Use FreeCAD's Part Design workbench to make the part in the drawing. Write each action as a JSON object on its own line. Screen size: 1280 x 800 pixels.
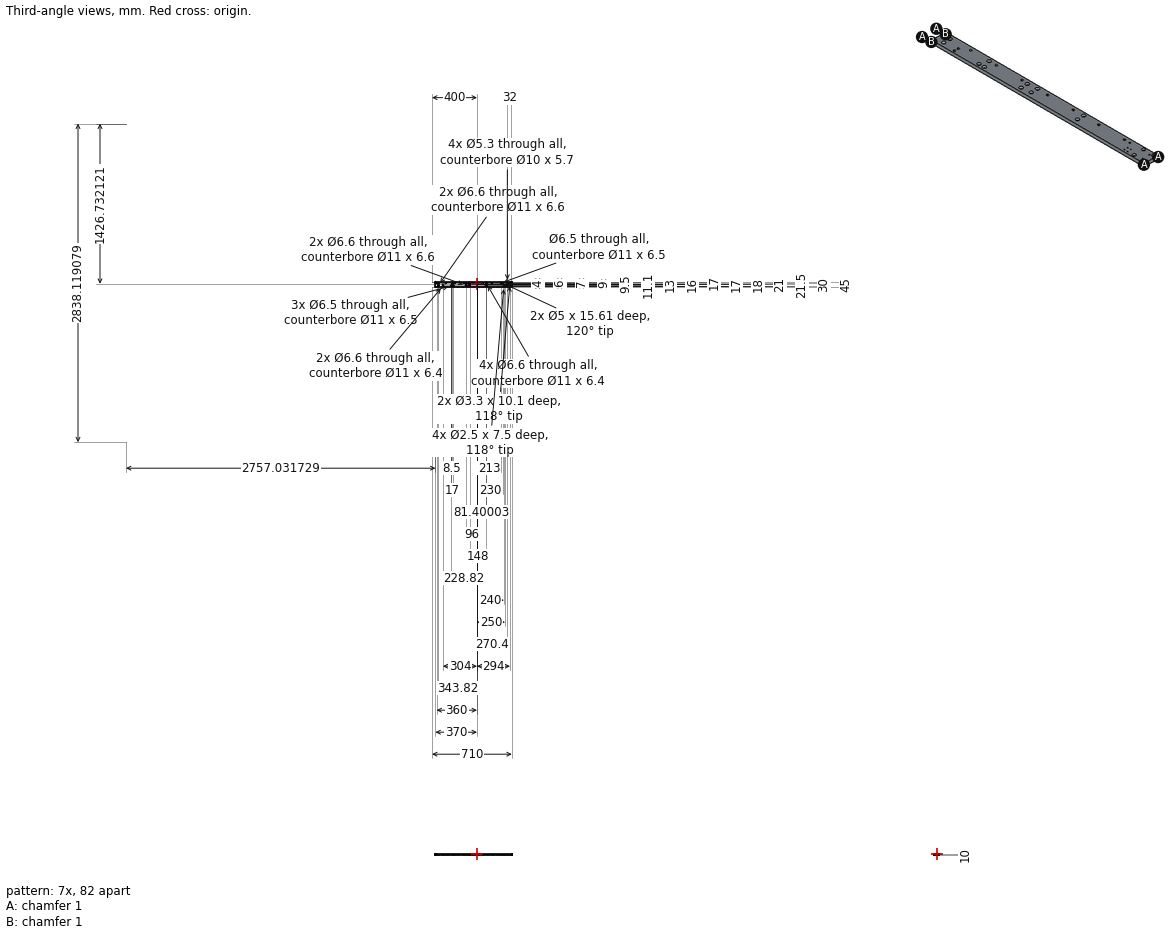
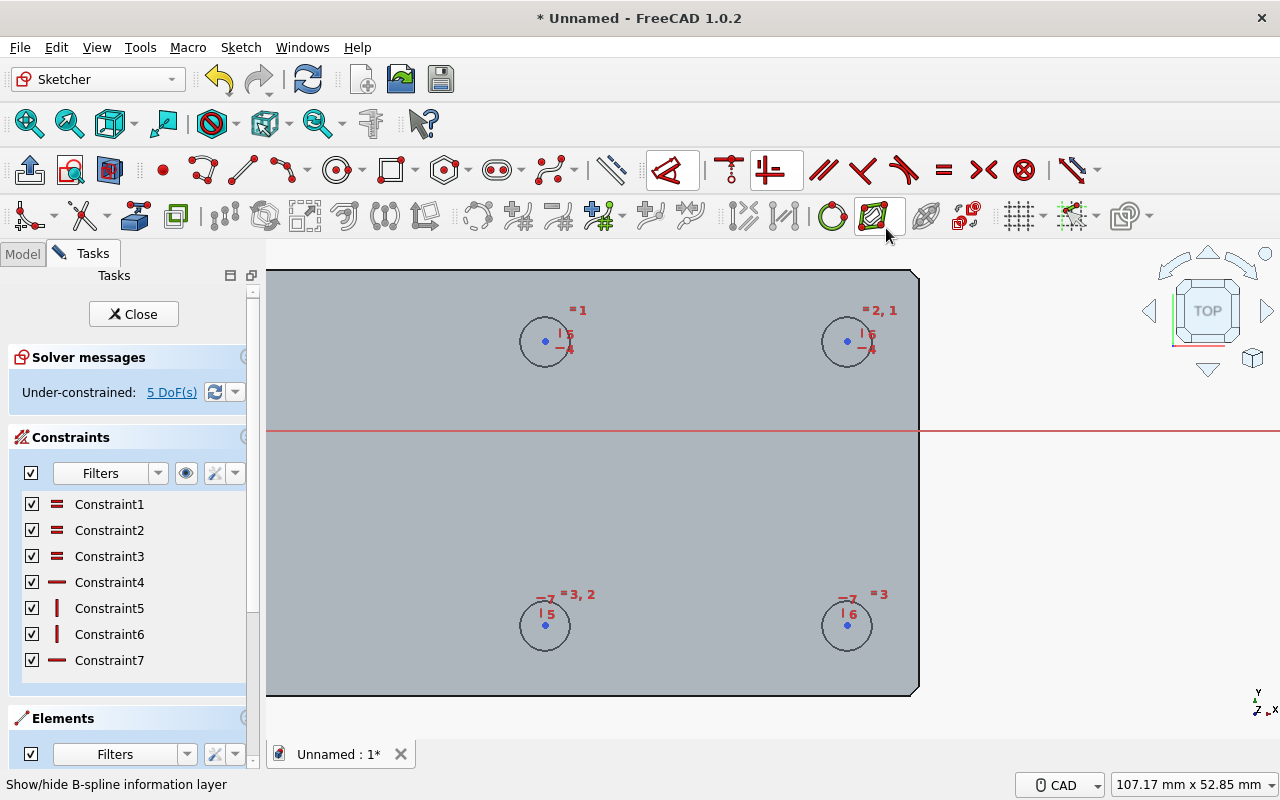
{"action": "left_click", "coordinate": [562, 324]}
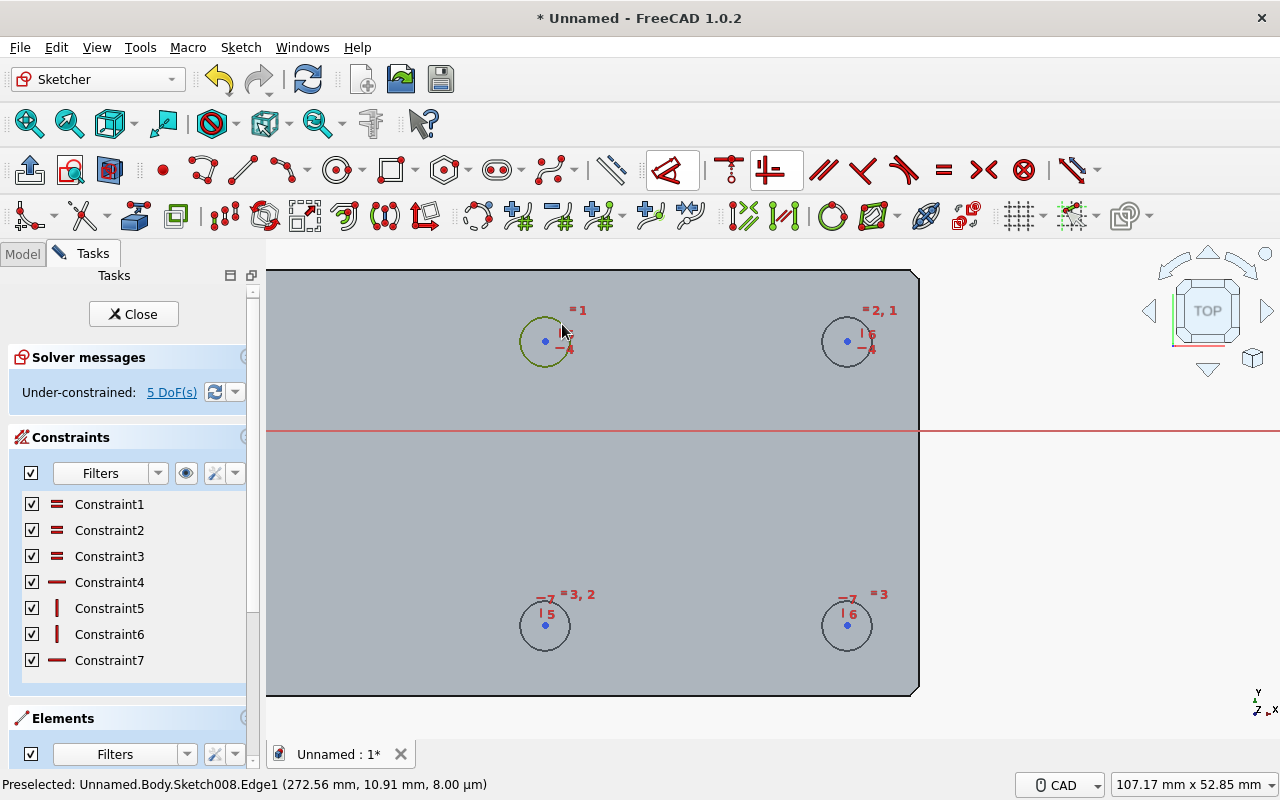
{"action": "key", "text": "k o"}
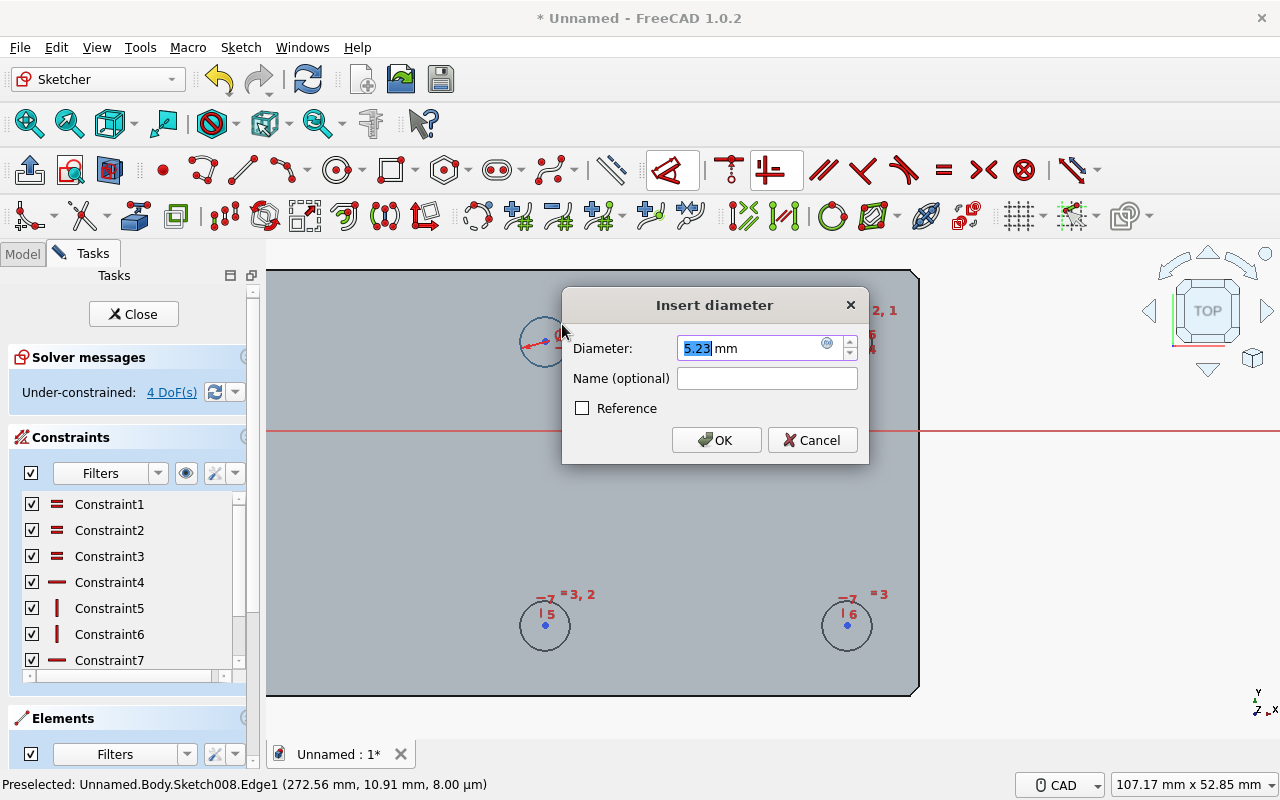
{"action": "type", "text": "5.3"}
{"action": "key", "text": "Return"}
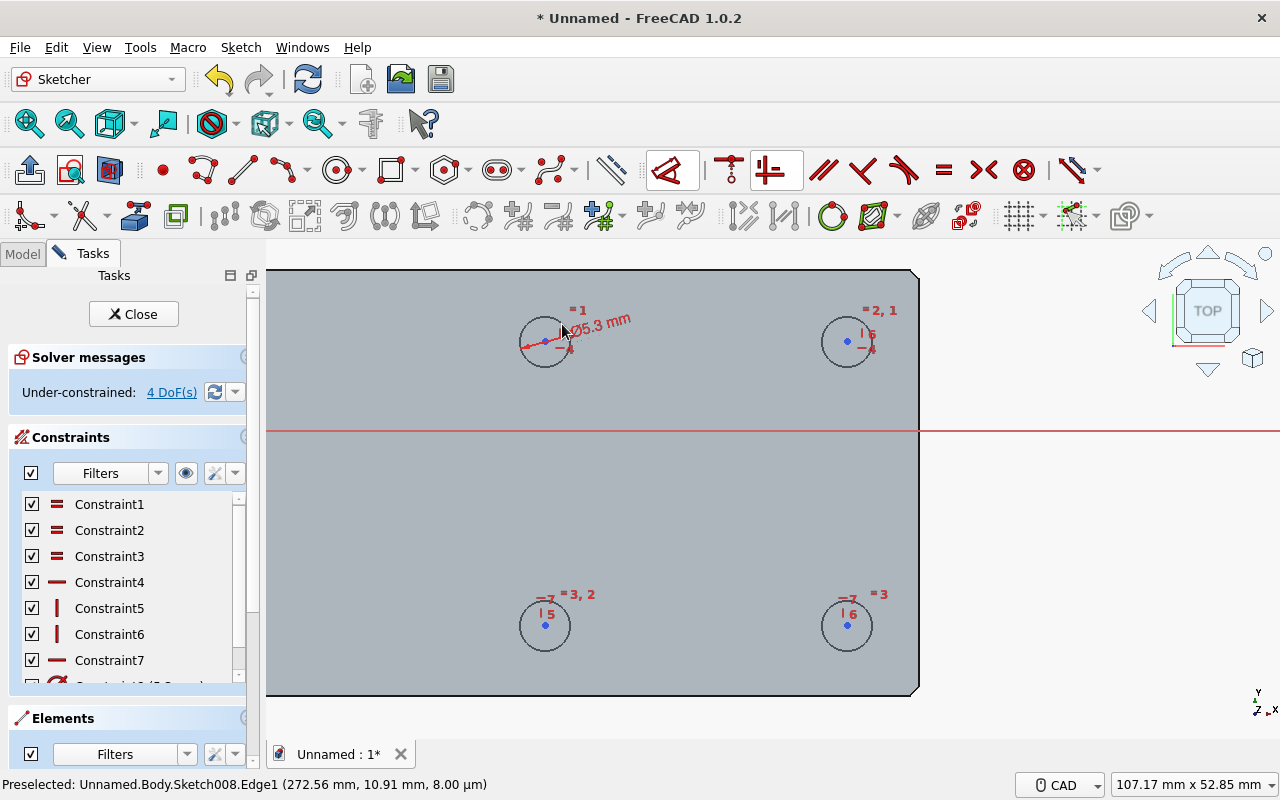
{"action": "left_click", "coordinate": [545, 342]}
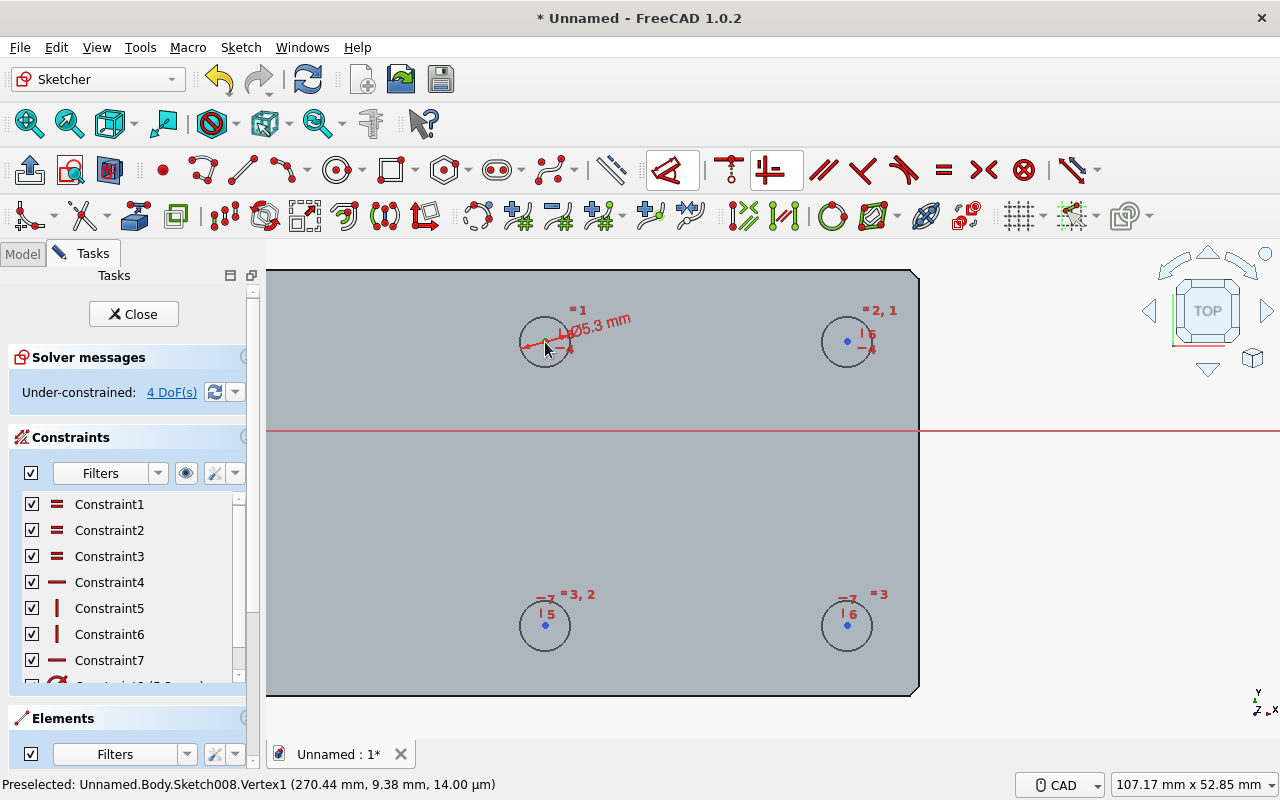
{"action": "left_click", "coordinate": [694, 170]}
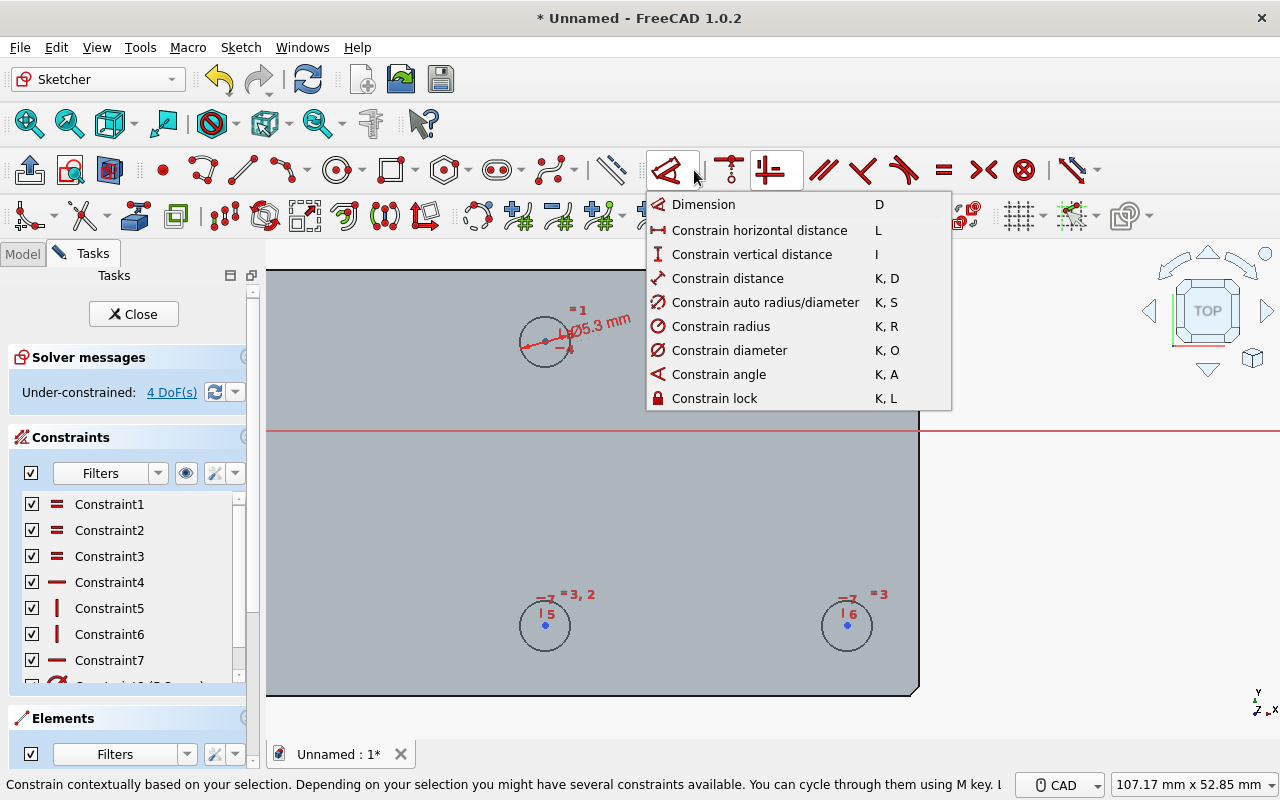
{"action": "left_click", "coordinate": [799, 254]}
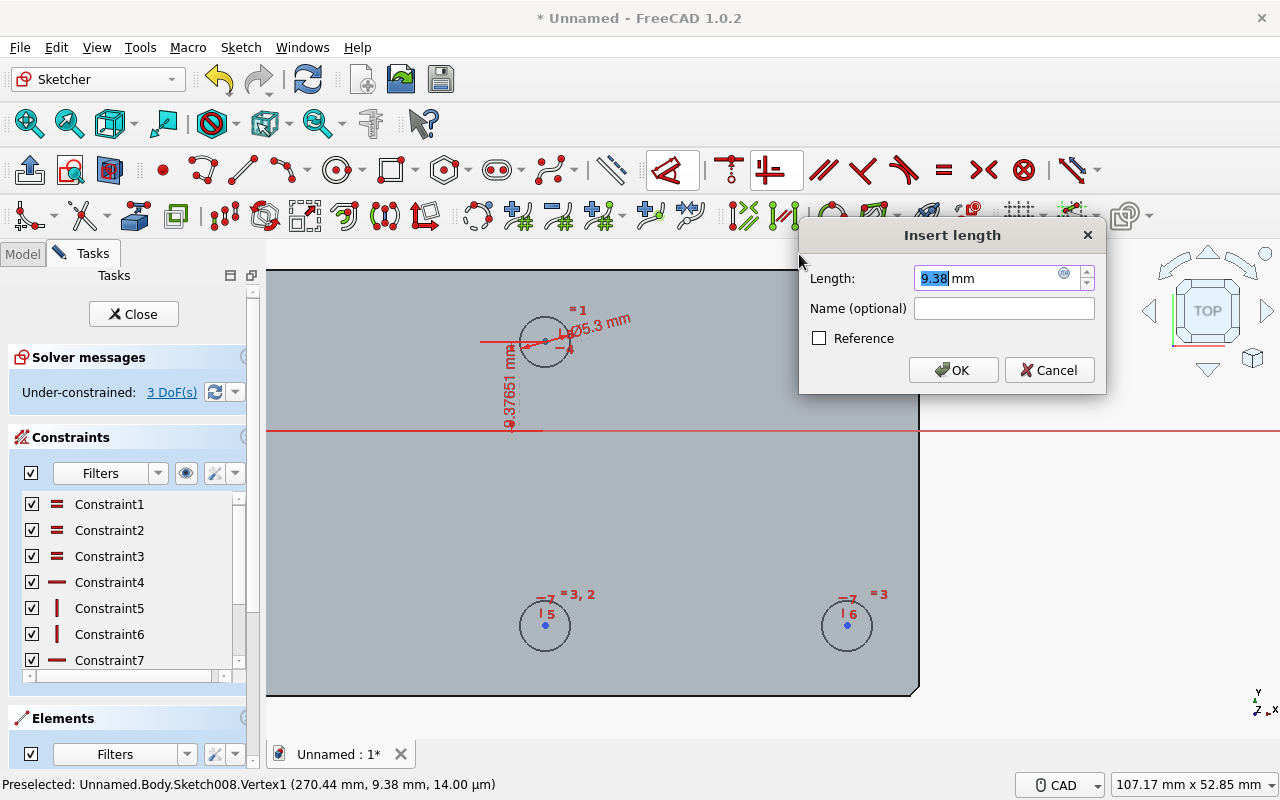
{"action": "type", "text": "9.5"}
{"action": "key", "text": "Return"}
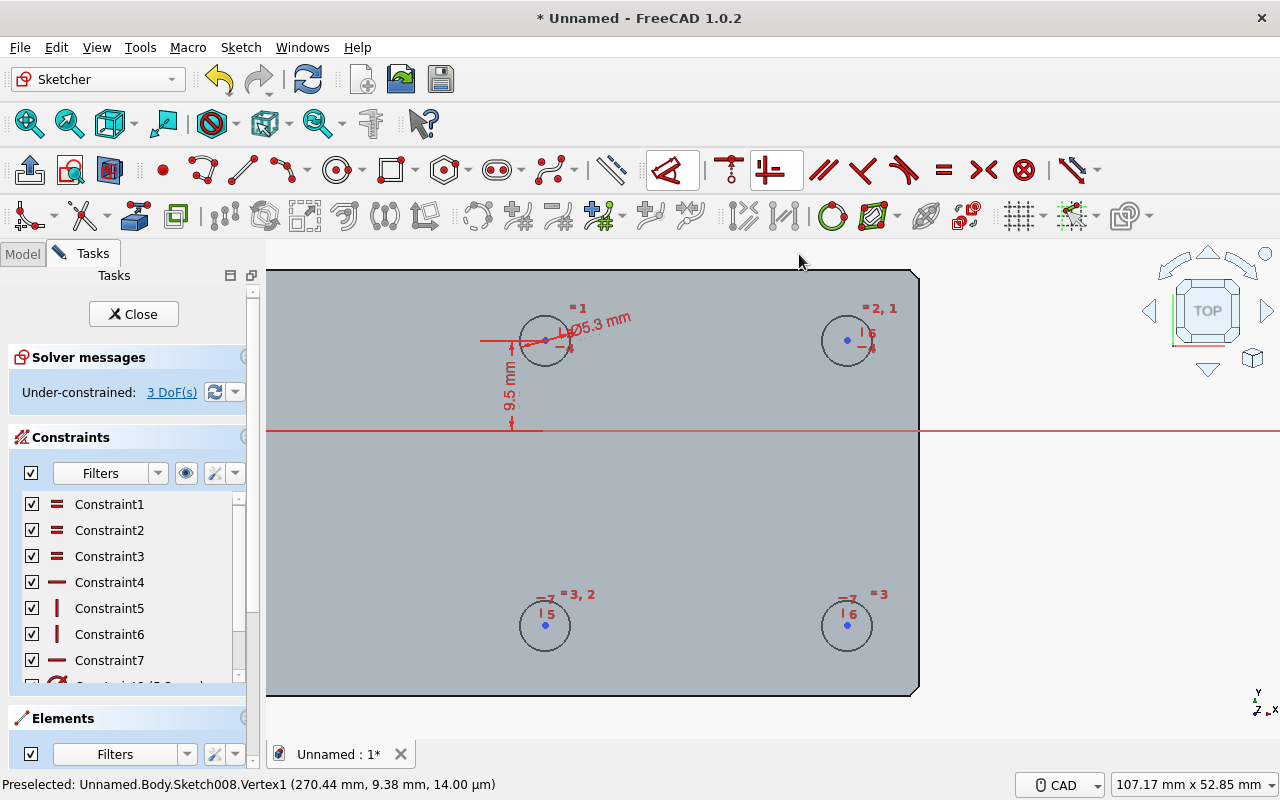
{"action": "left_click", "coordinate": [545, 341]}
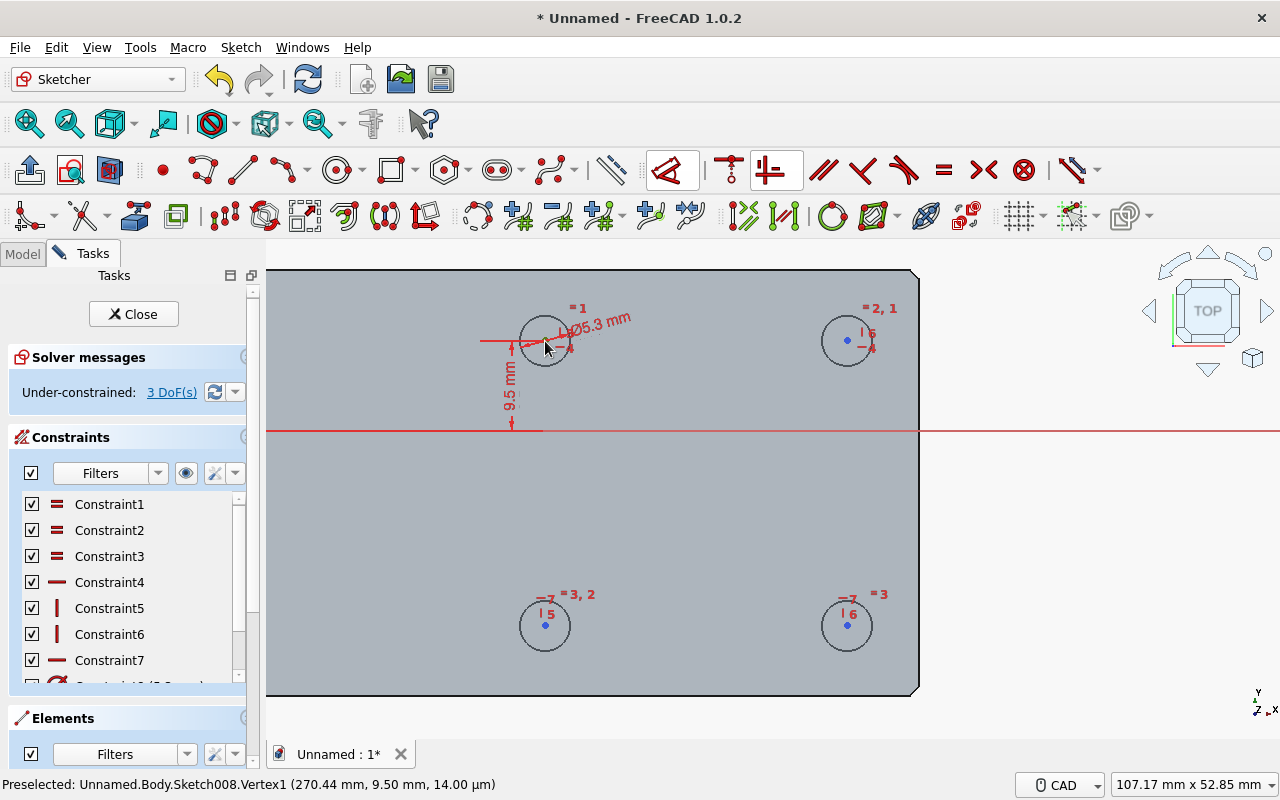
{"action": "left_click", "coordinate": [847, 341]}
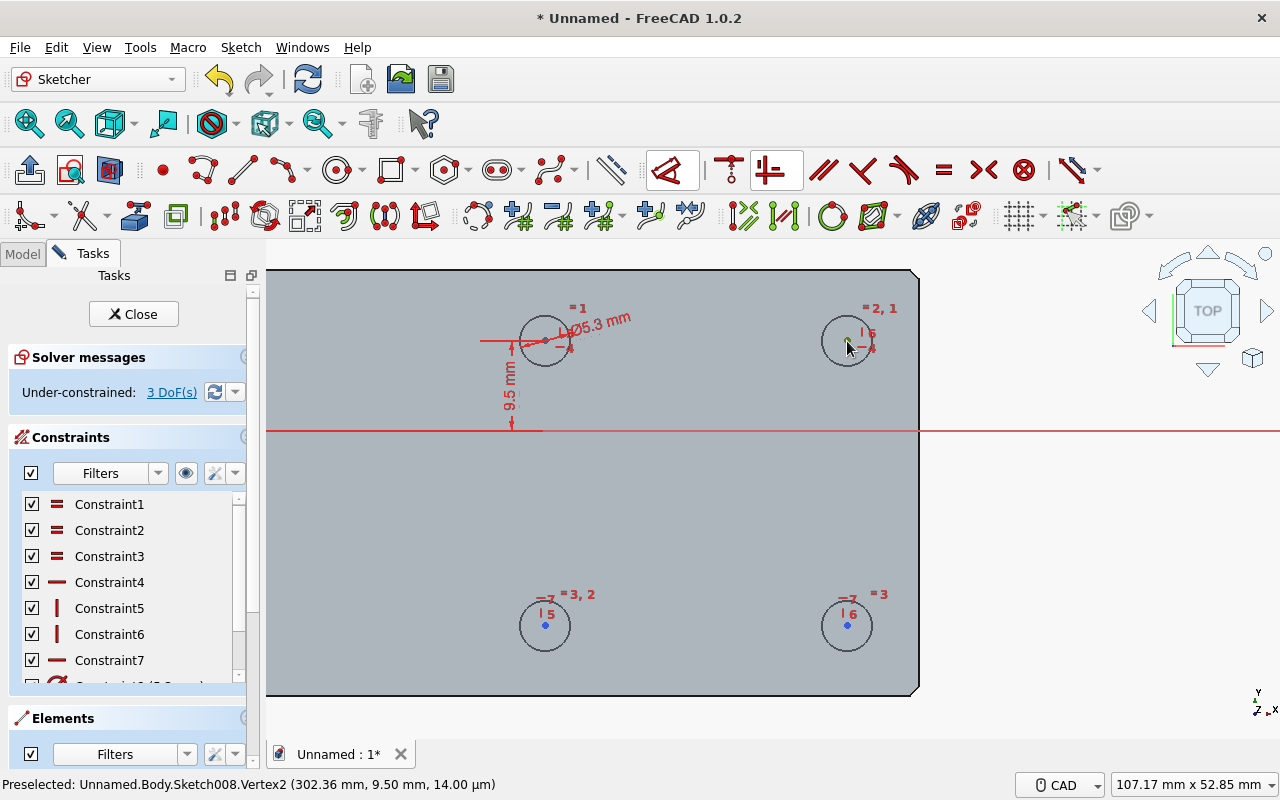
{"action": "key", "text": "l"}